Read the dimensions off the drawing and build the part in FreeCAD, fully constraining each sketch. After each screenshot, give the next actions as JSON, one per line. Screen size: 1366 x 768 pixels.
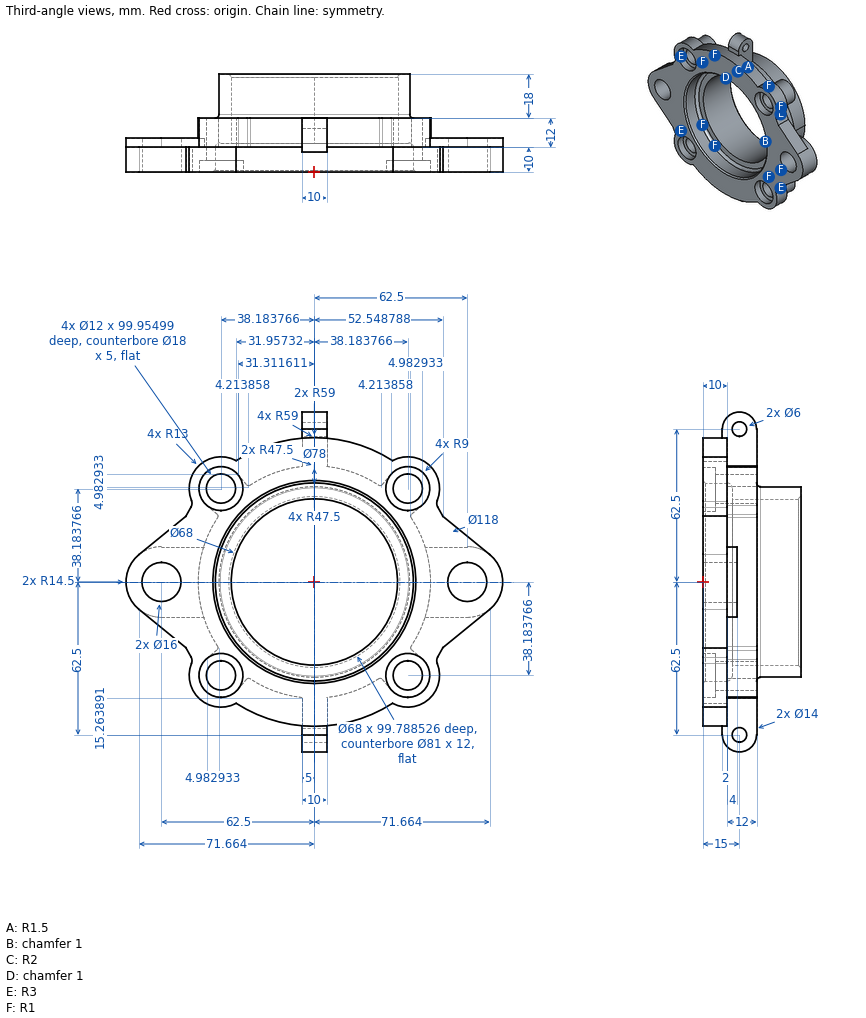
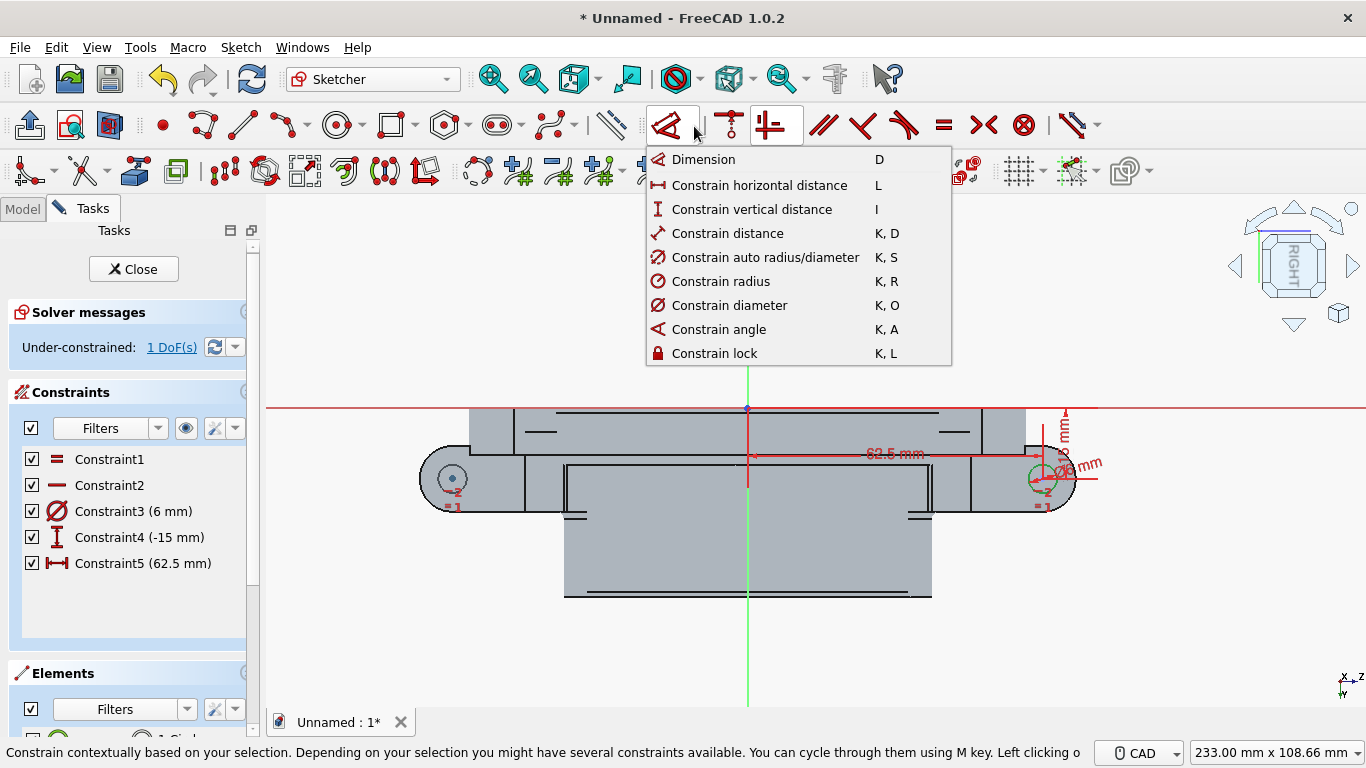
{"action": "left_click", "coordinate": [799, 185]}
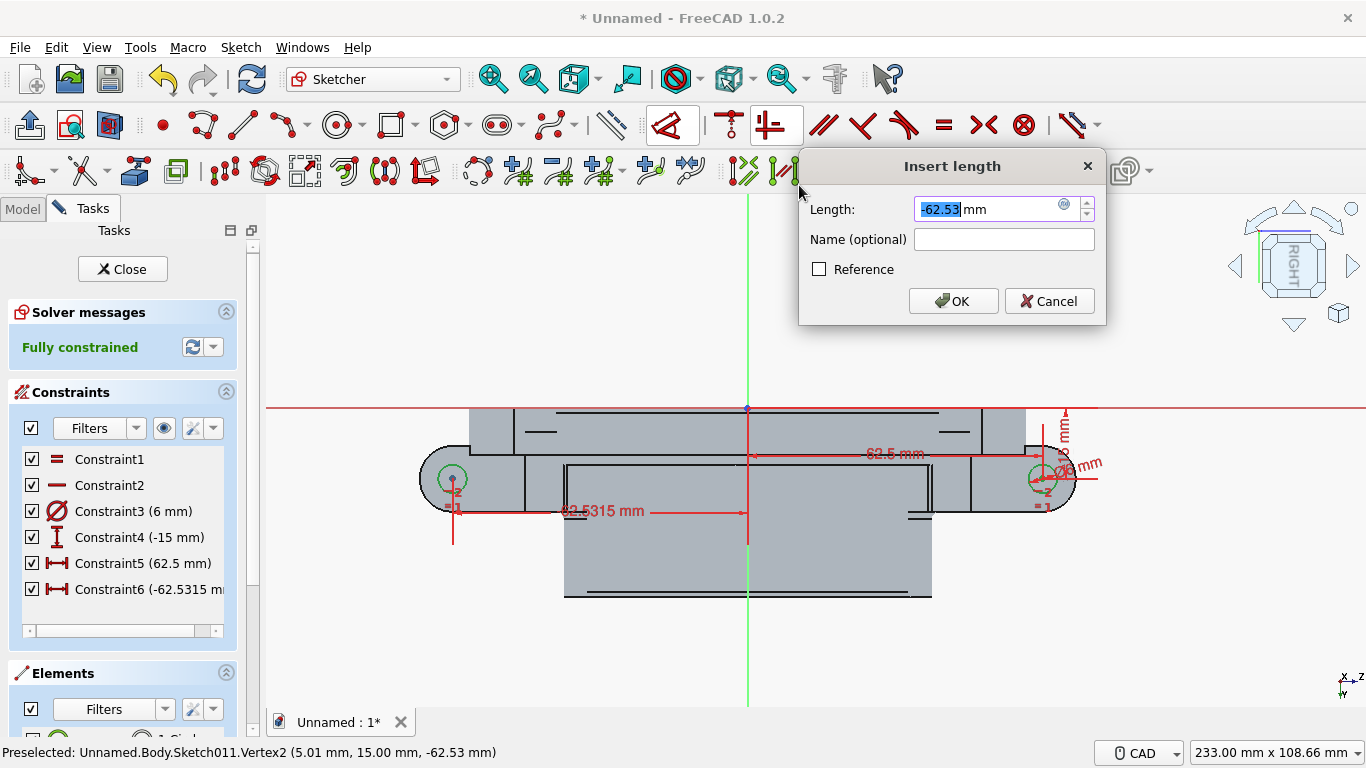
{"action": "type", "text": "-62.5"}
{"action": "key", "text": "Return"}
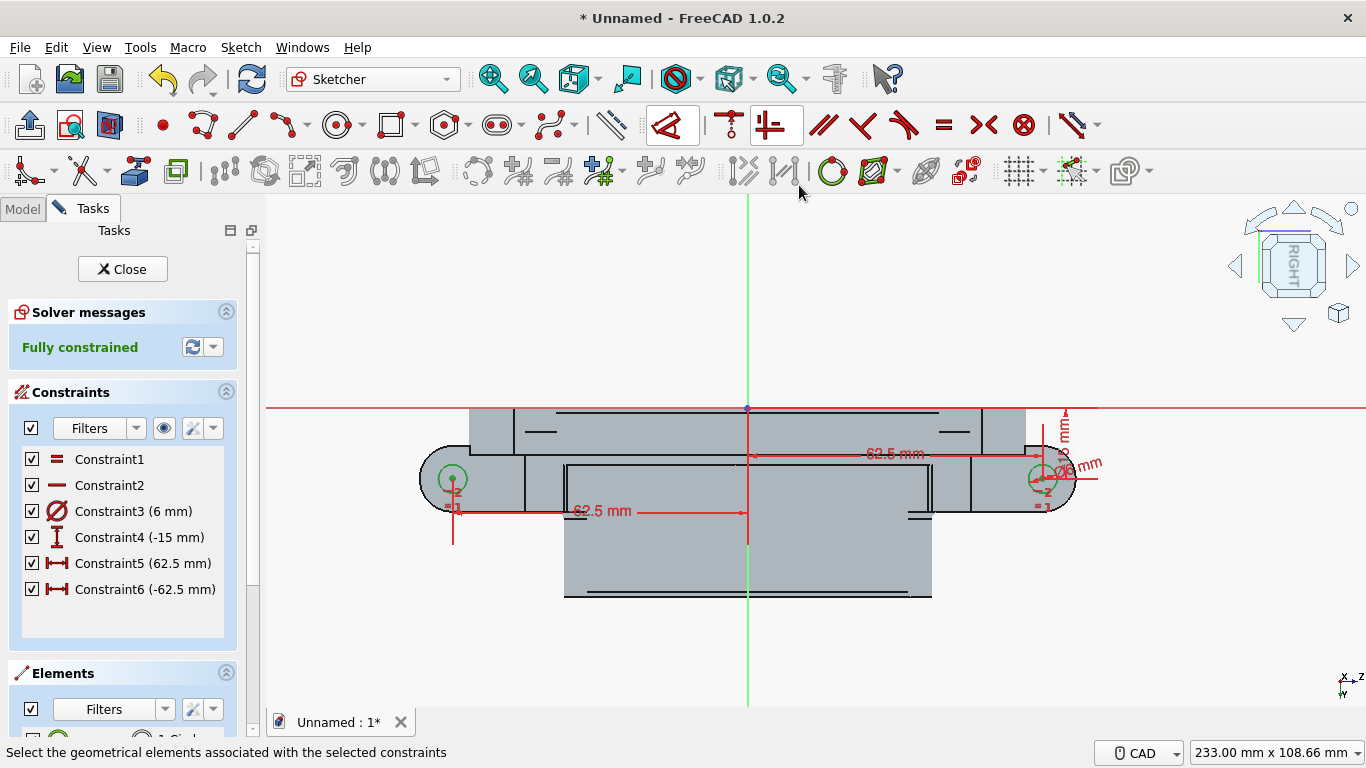
{"action": "left_click", "coordinate": [123, 269]}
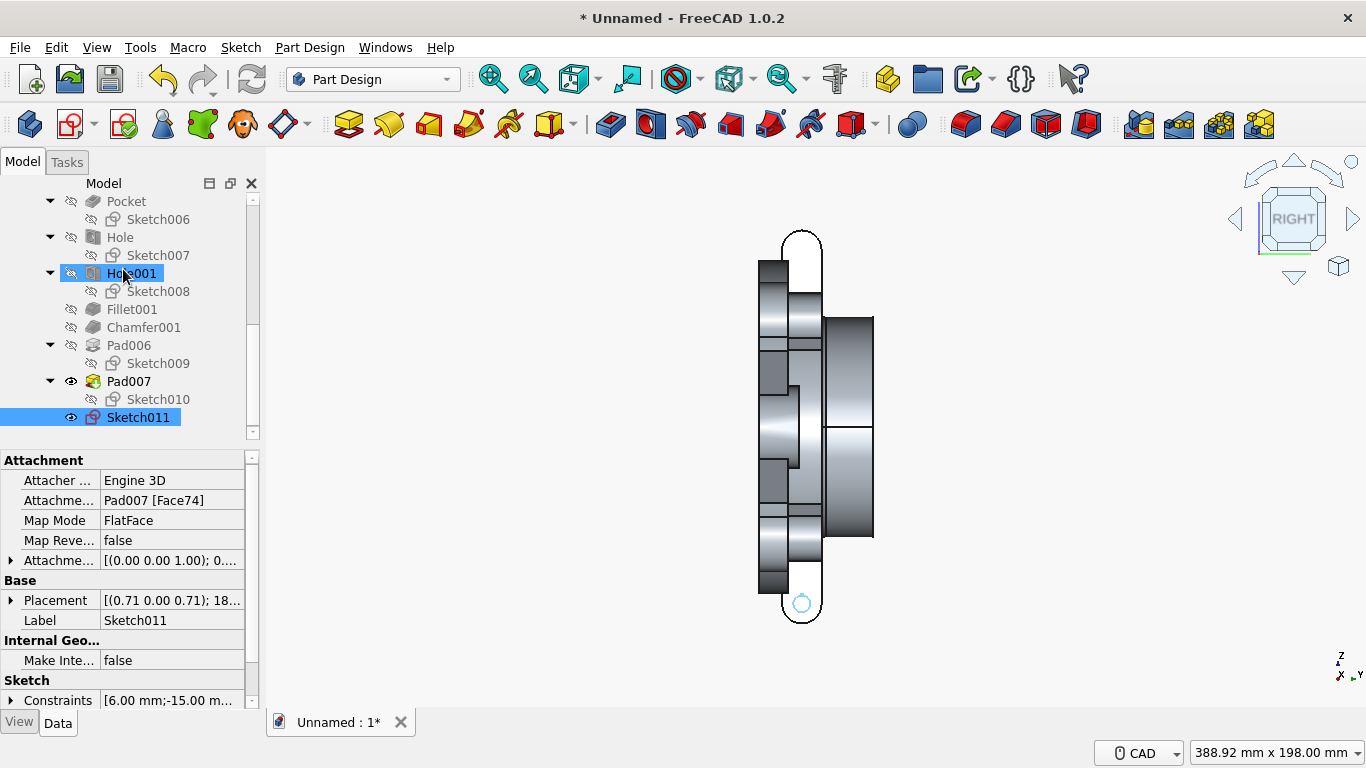
{"action": "left_click", "coordinate": [612, 124]}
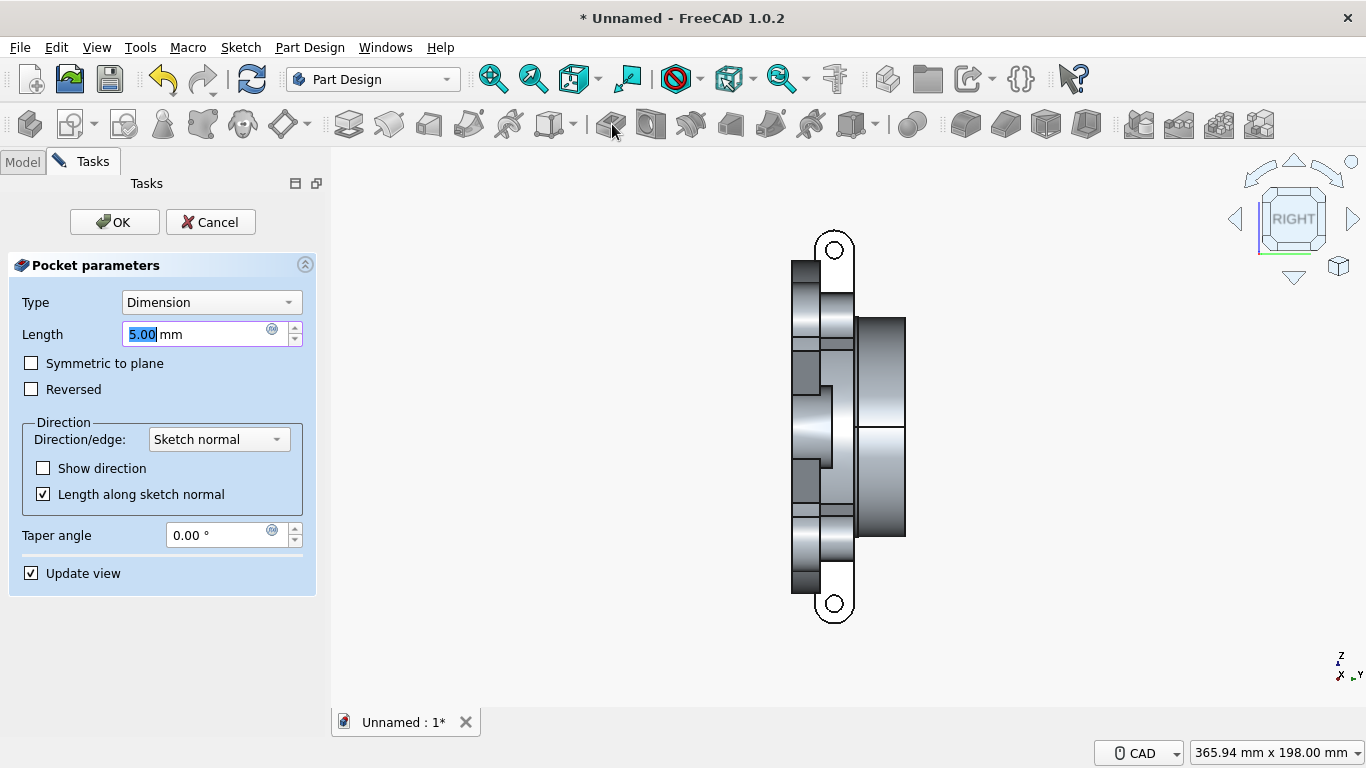
{"action": "type", "text": "10"}
{"action": "key", "text": "Tab"}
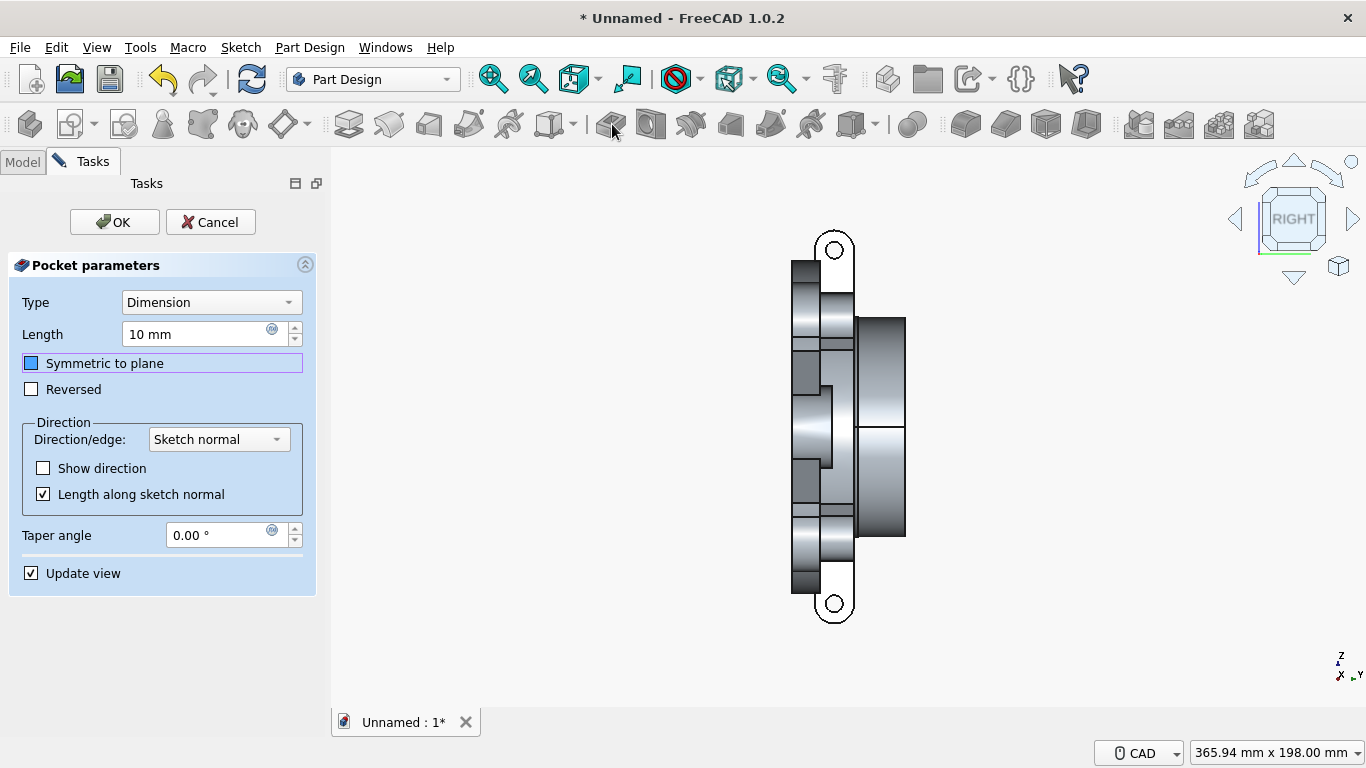
{"action": "left_click", "coordinate": [115, 222]}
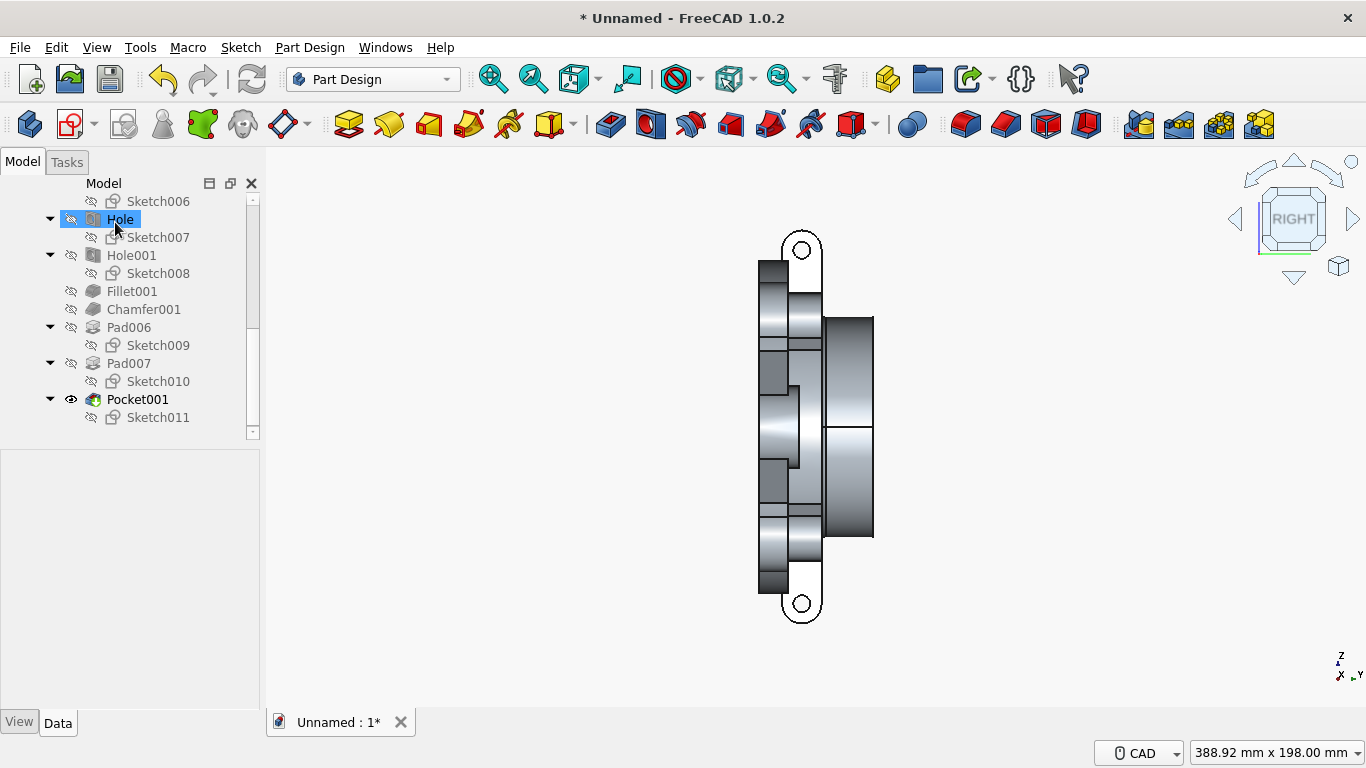
{"action": "key", "text": "0"}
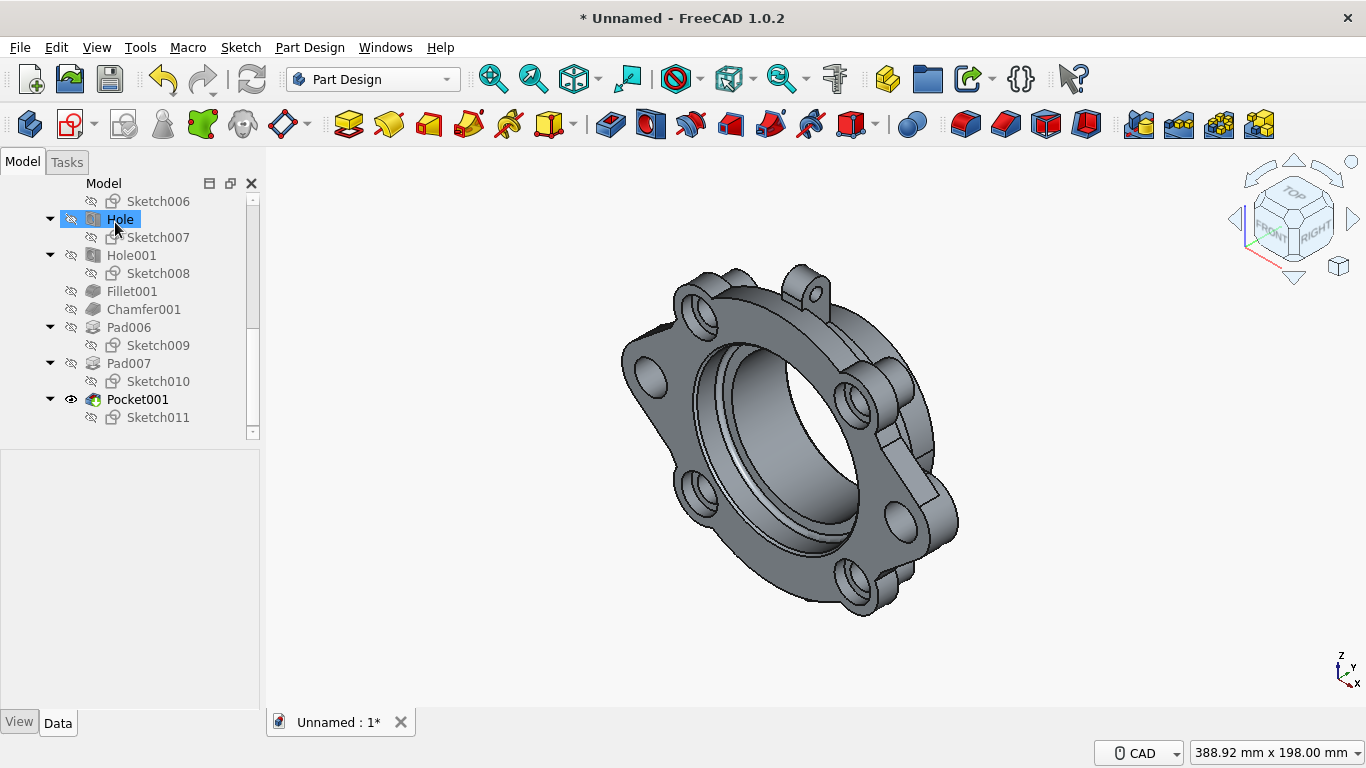
{"action": "key", "text": "2"}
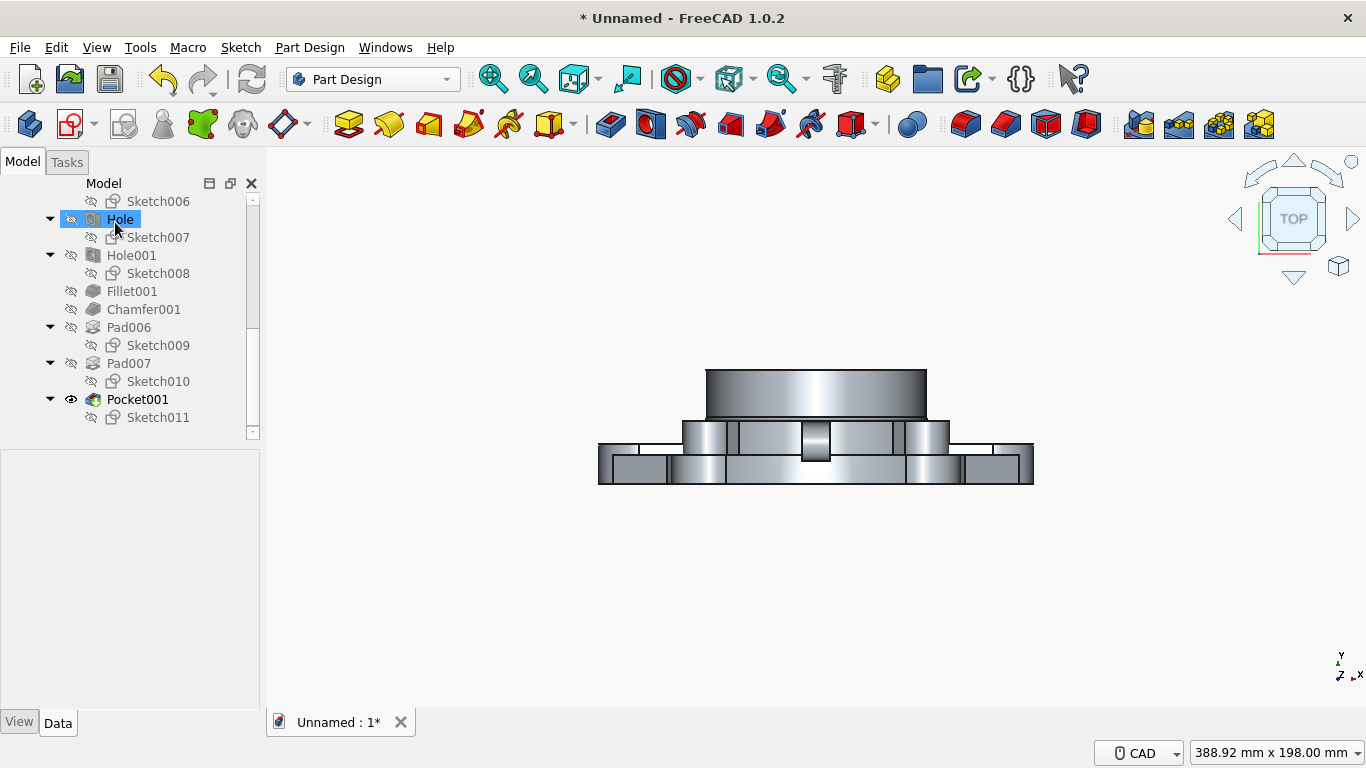
{"action": "left_click", "coordinate": [494, 80]}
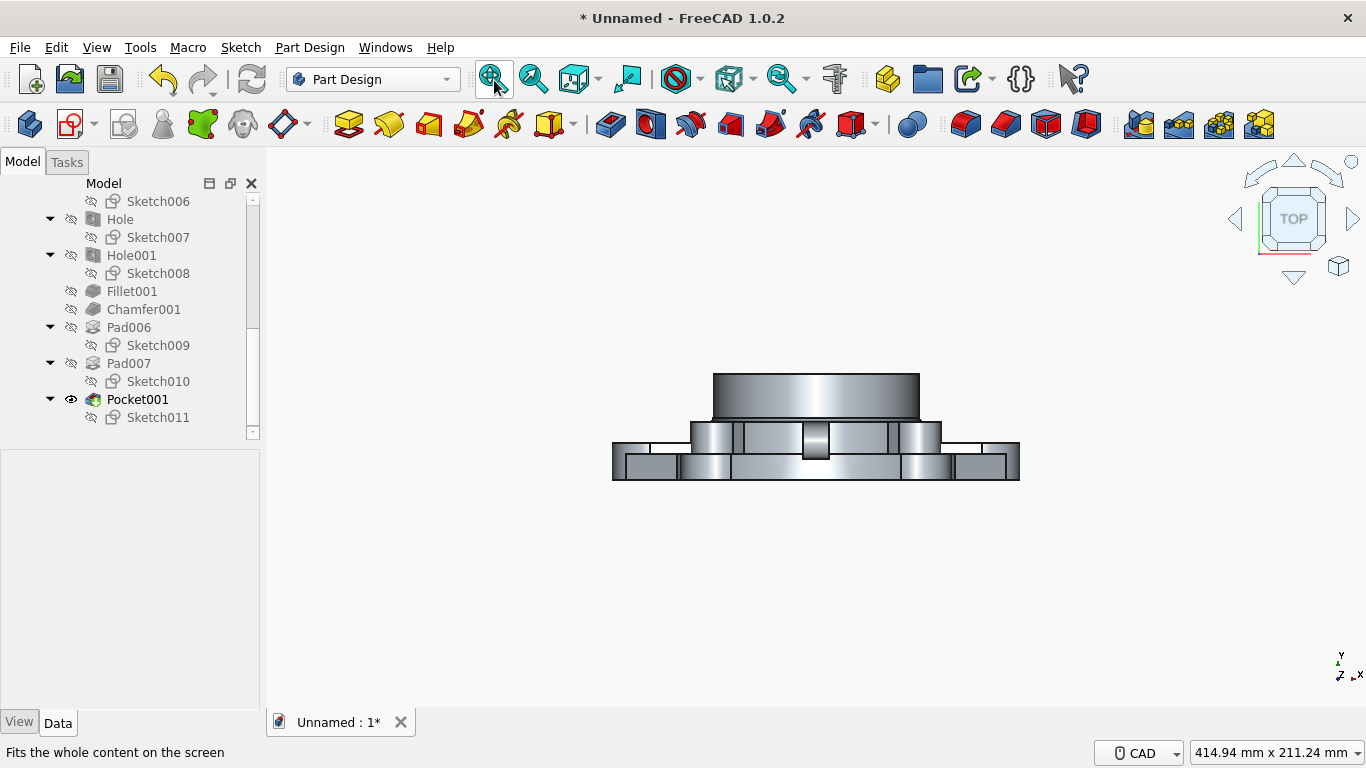
{"action": "key", "text": "1"}